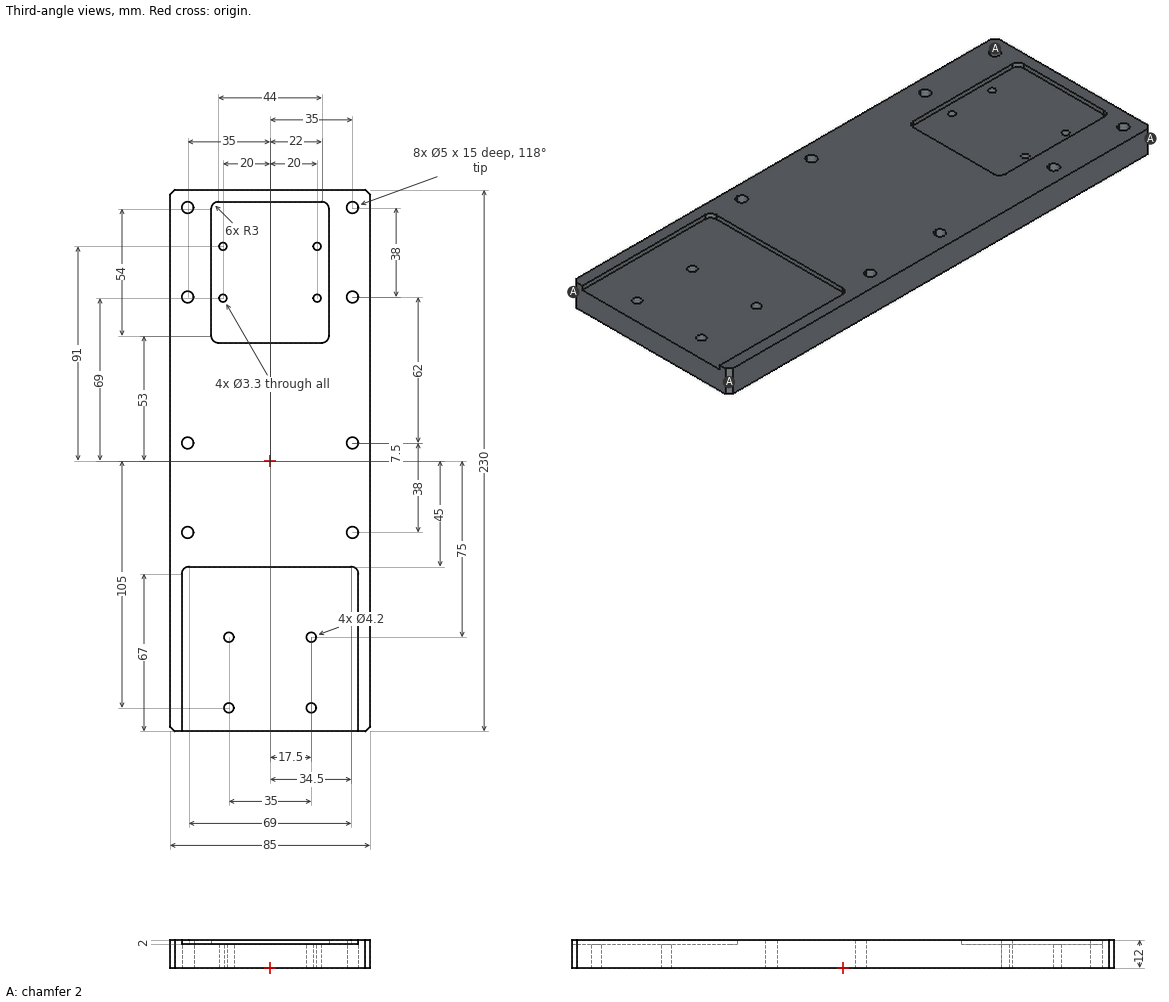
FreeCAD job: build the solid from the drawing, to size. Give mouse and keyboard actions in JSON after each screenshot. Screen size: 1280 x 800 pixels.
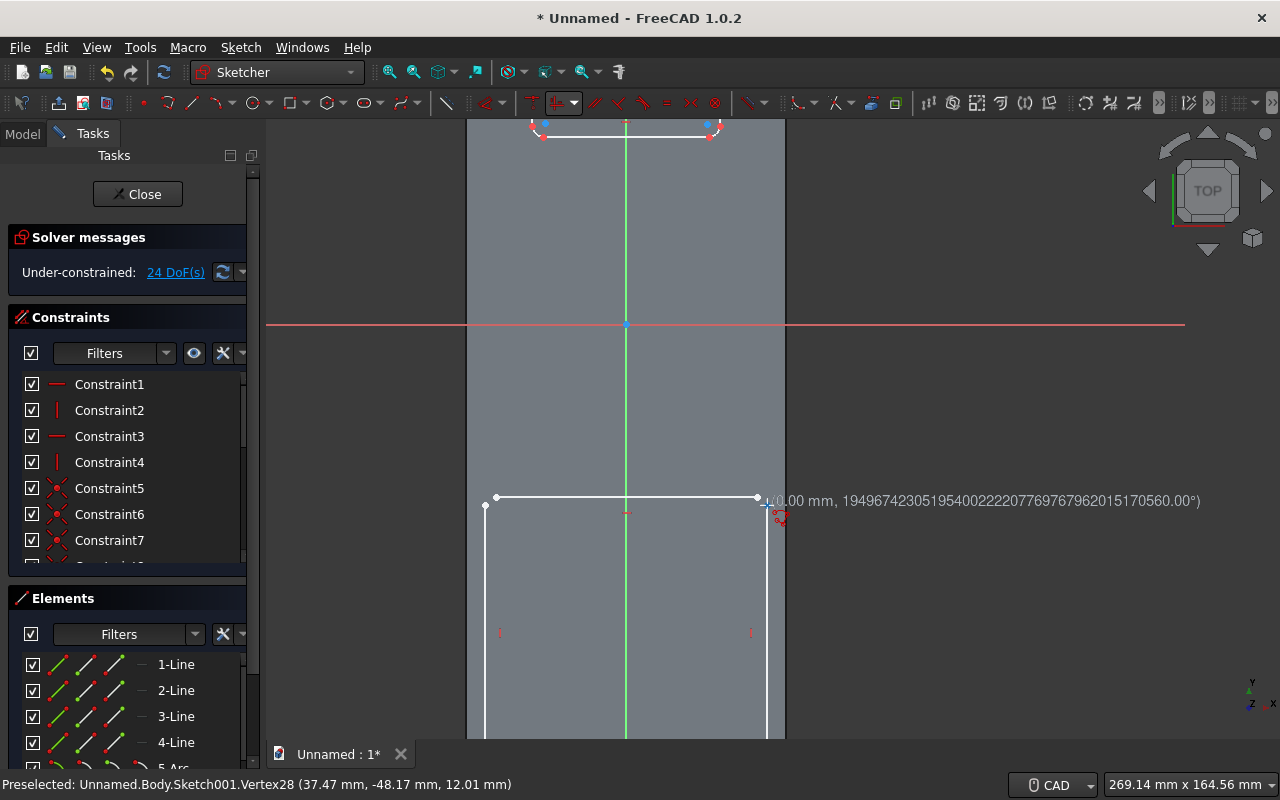
{"action": "key", "text": "g 3 a"}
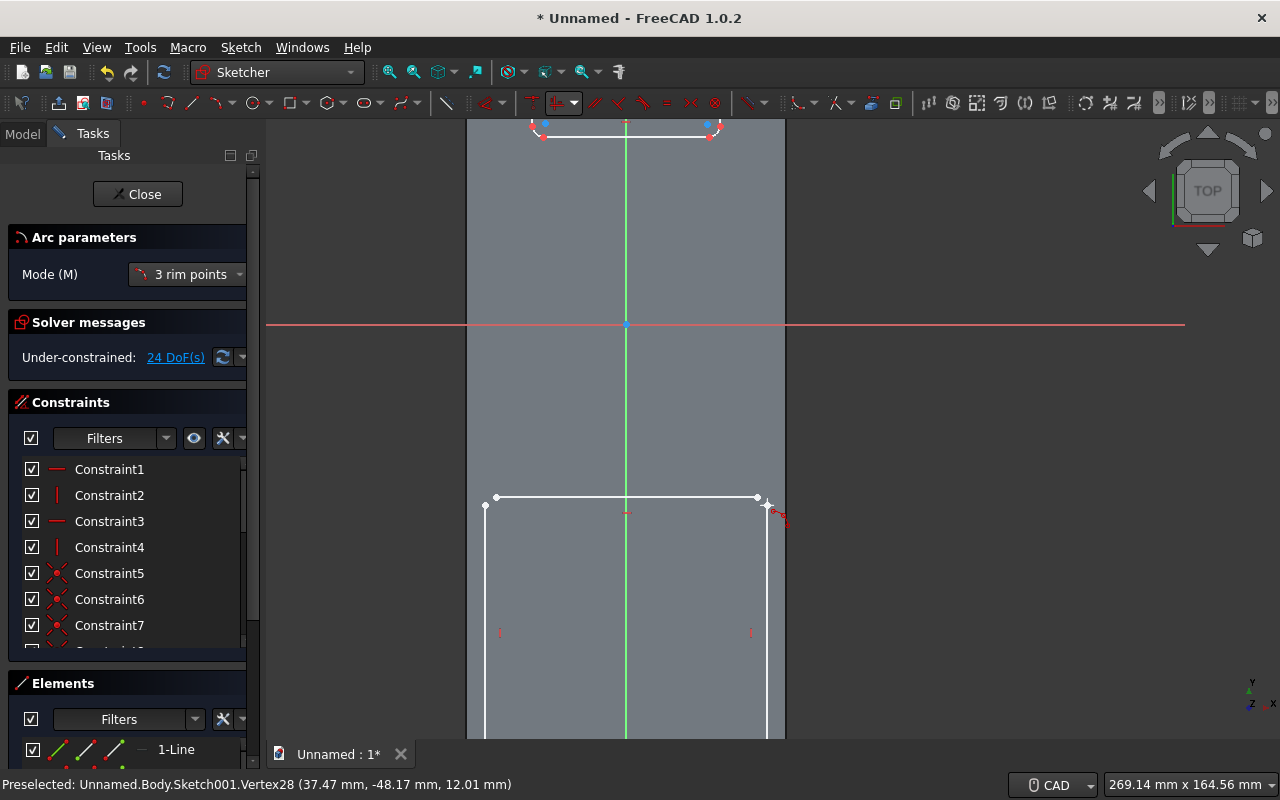
{"action": "left_click", "coordinate": [497, 497]}
{"action": "left_click", "coordinate": [485, 506]}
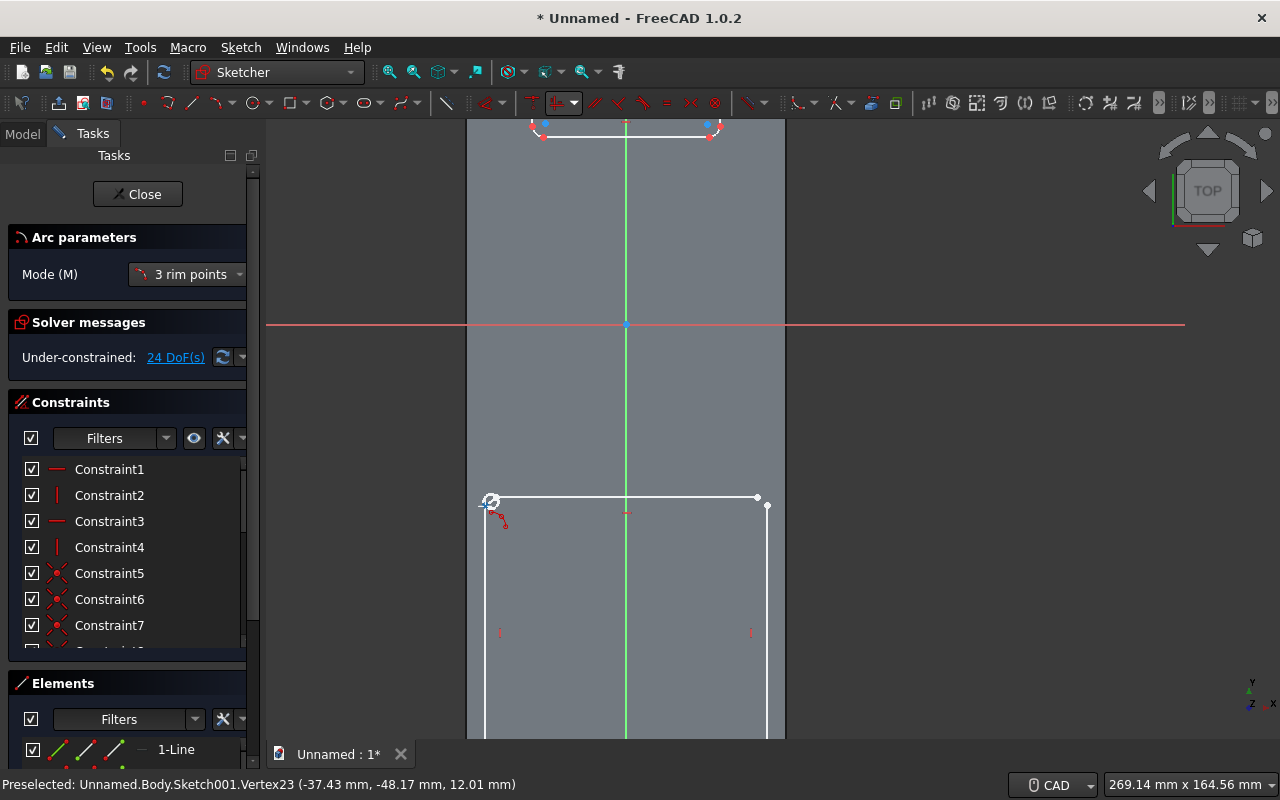
{"action": "scroll", "coordinate": [488, 497], "scroll_direction": "up", "scroll_amount": 8}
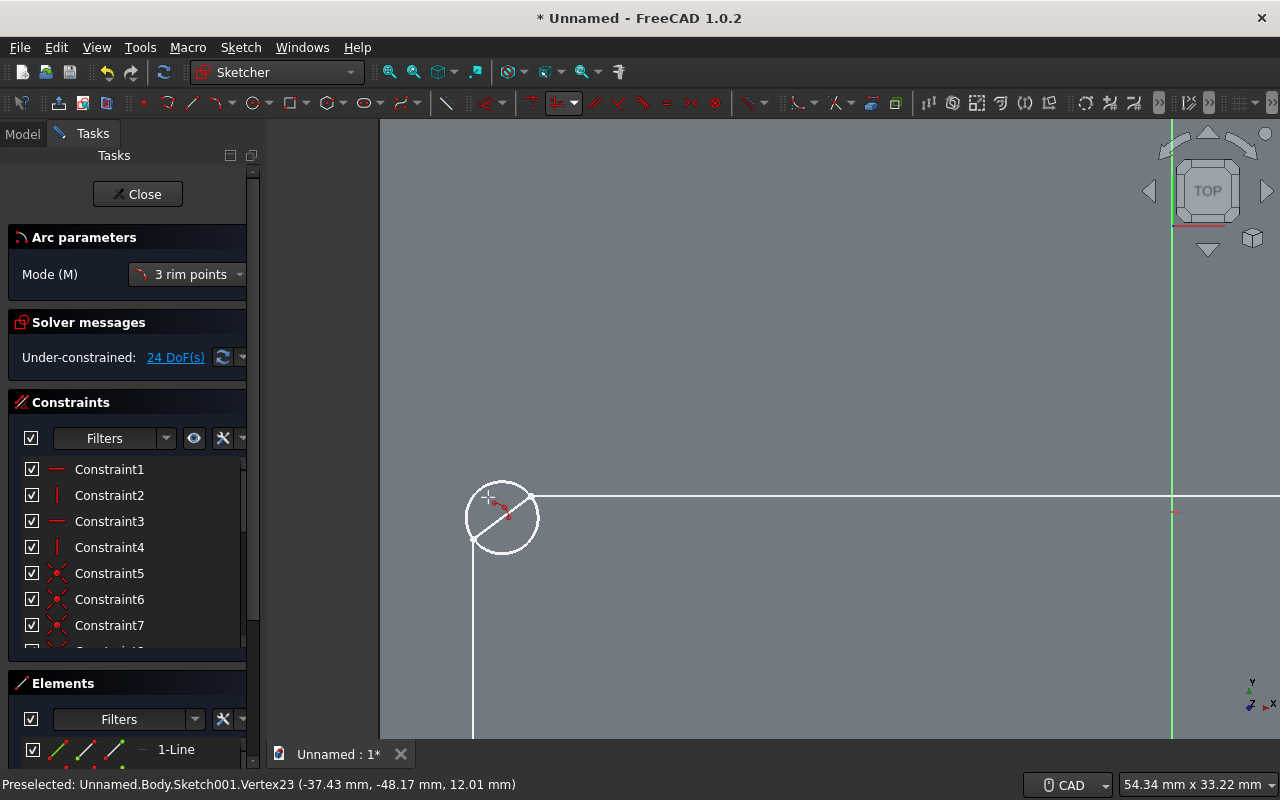
{"action": "left_click", "coordinate": [488, 496]}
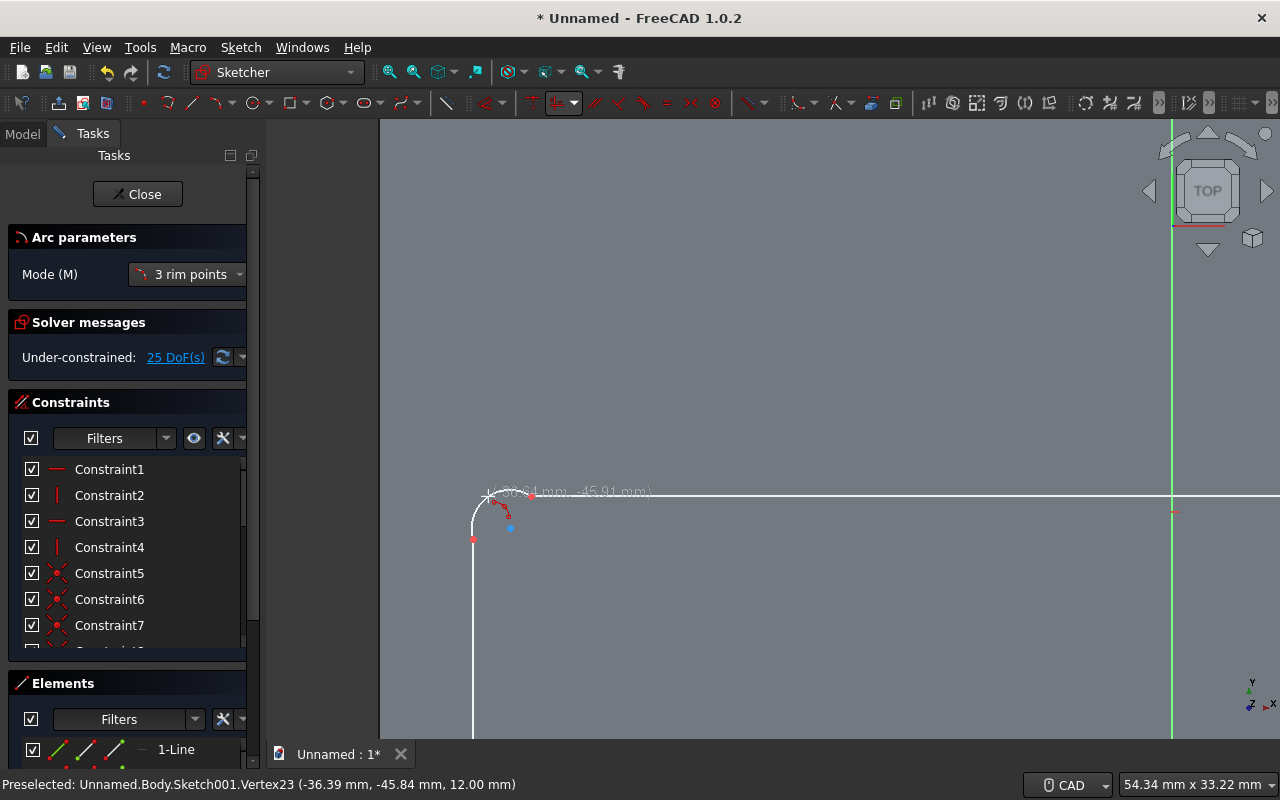
{"action": "scroll", "coordinate": [658, 503], "scroll_direction": "down", "scroll_amount": 12}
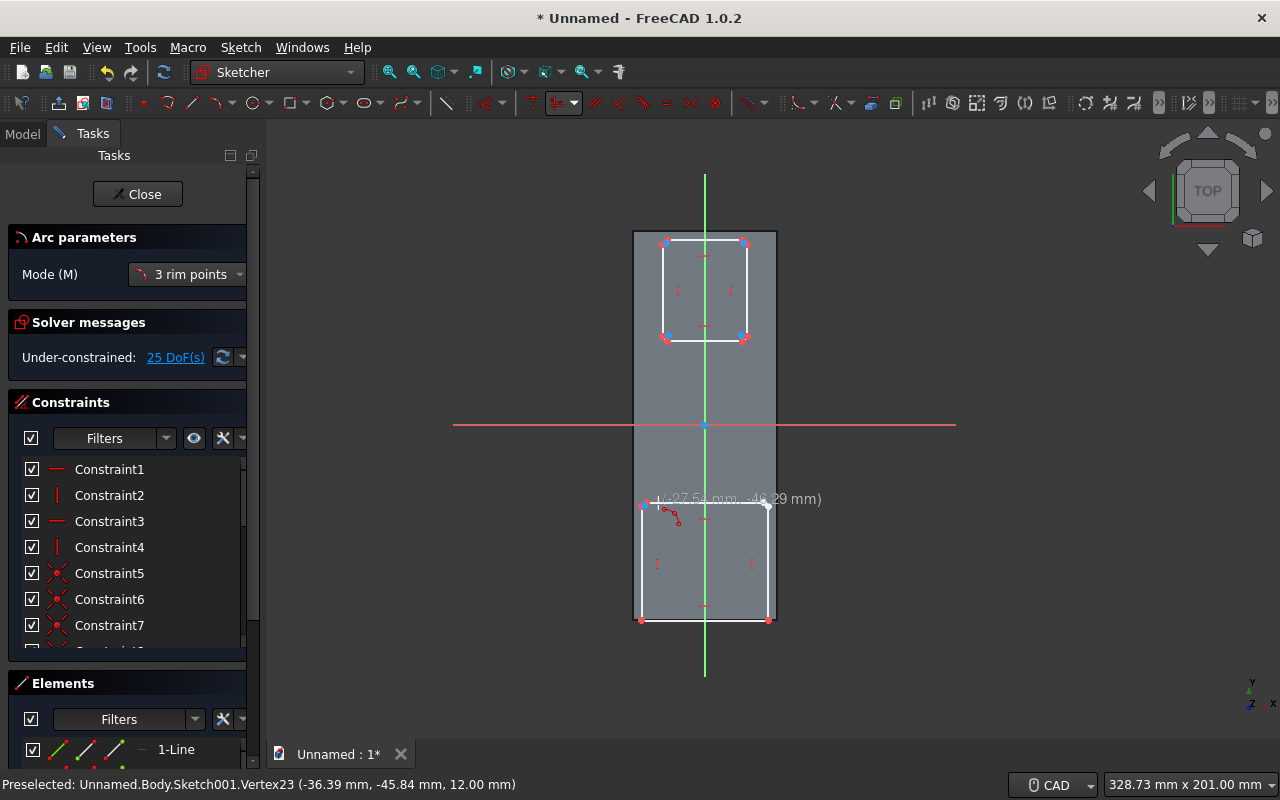
{"action": "scroll", "coordinate": [768, 507], "scroll_direction": "up", "scroll_amount": 4}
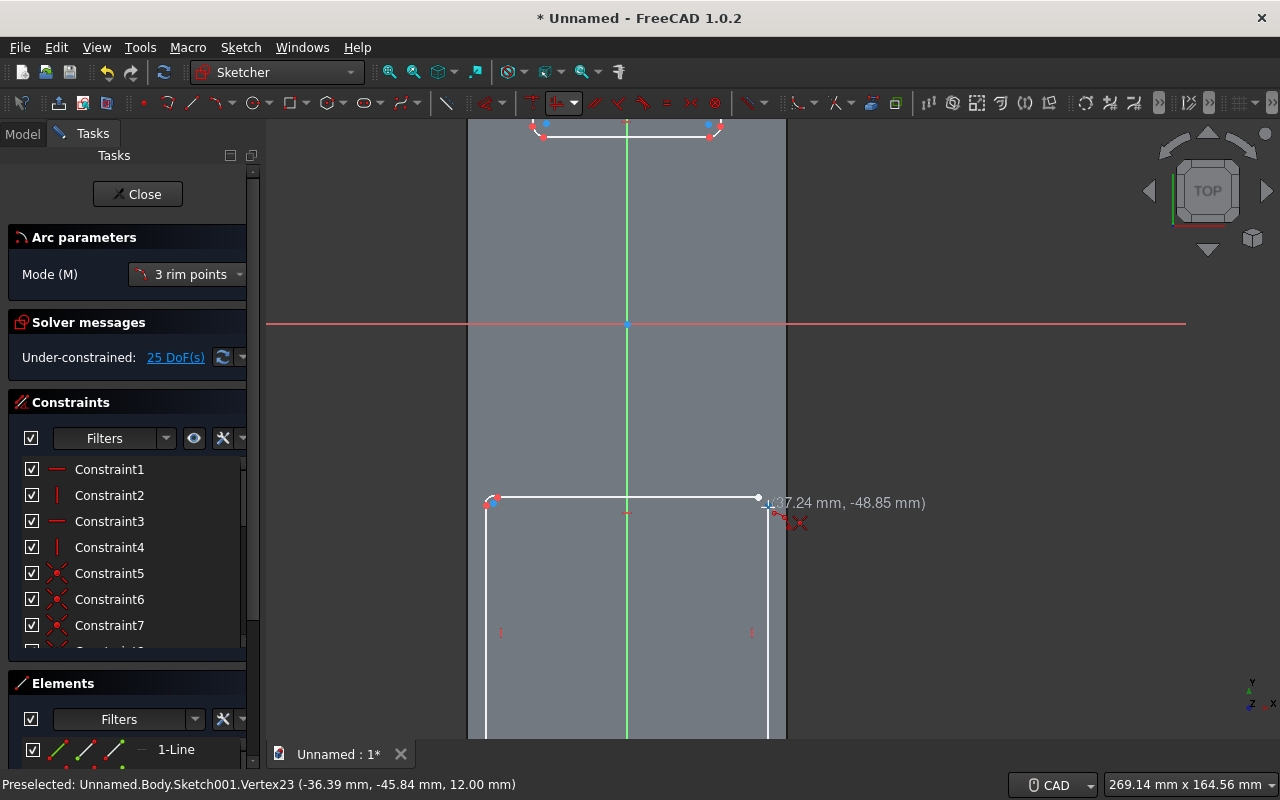
{"action": "left_click", "coordinate": [768, 506]}
{"action": "left_click", "coordinate": [758, 497]}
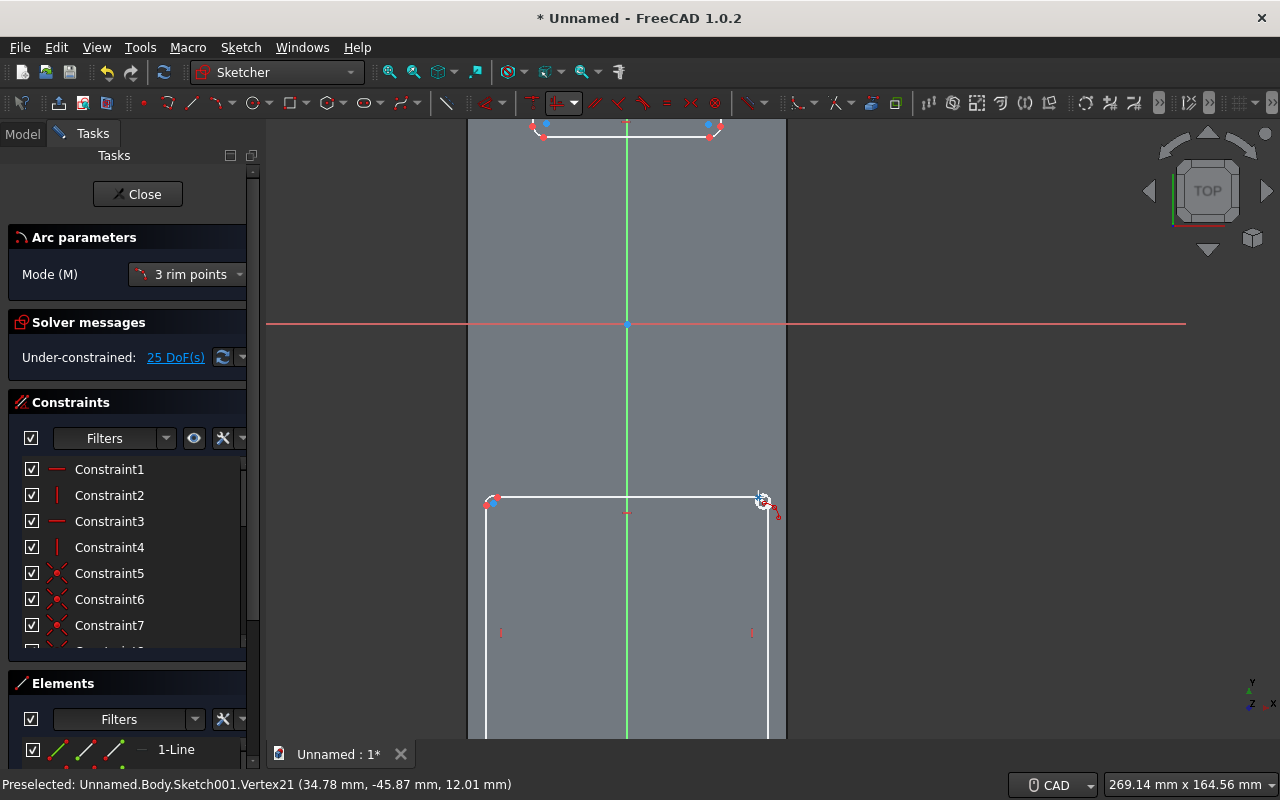
{"action": "scroll", "coordinate": [765, 497], "scroll_direction": "up", "scroll_amount": 8}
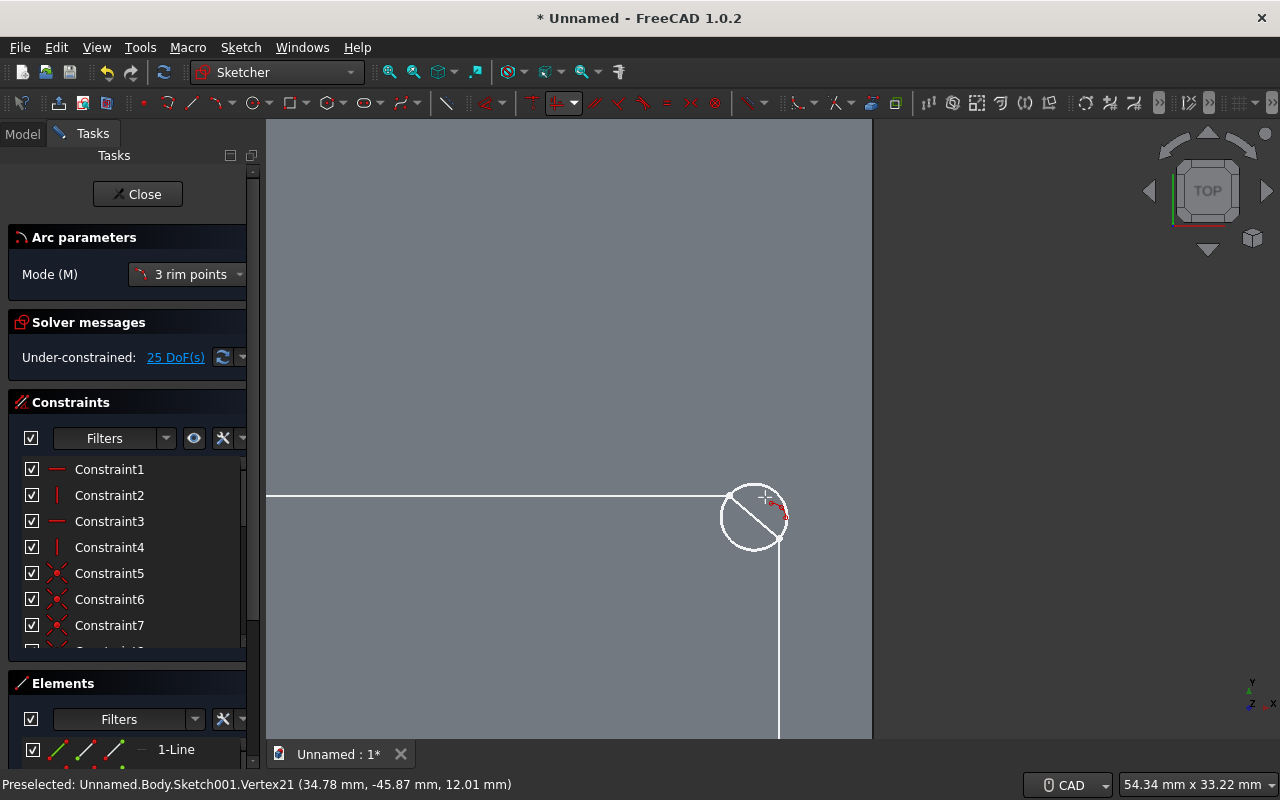
{"action": "left_click", "coordinate": [763, 496]}
{"action": "key", "text": "Escape"}